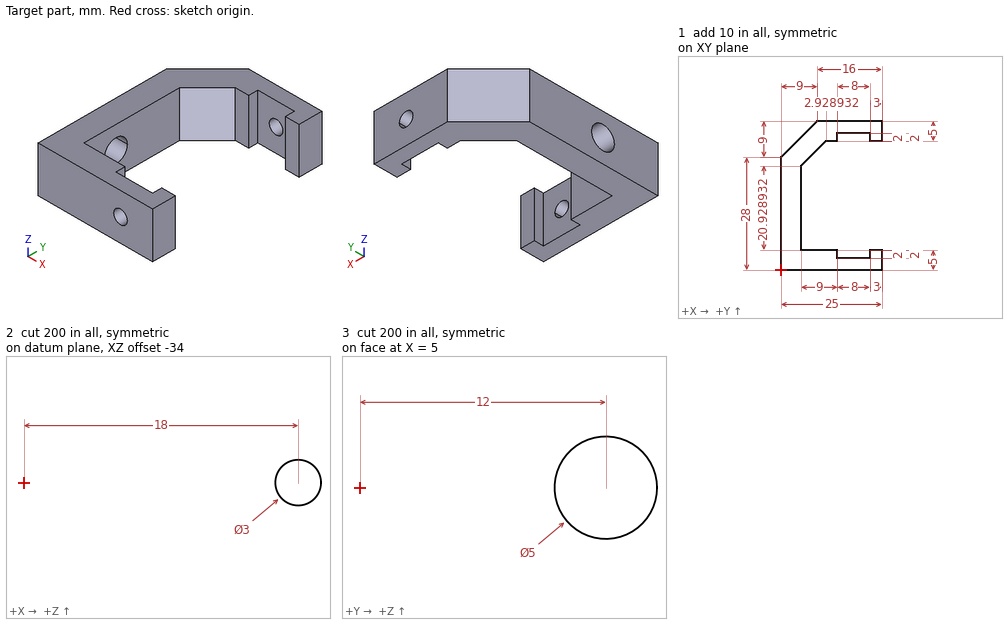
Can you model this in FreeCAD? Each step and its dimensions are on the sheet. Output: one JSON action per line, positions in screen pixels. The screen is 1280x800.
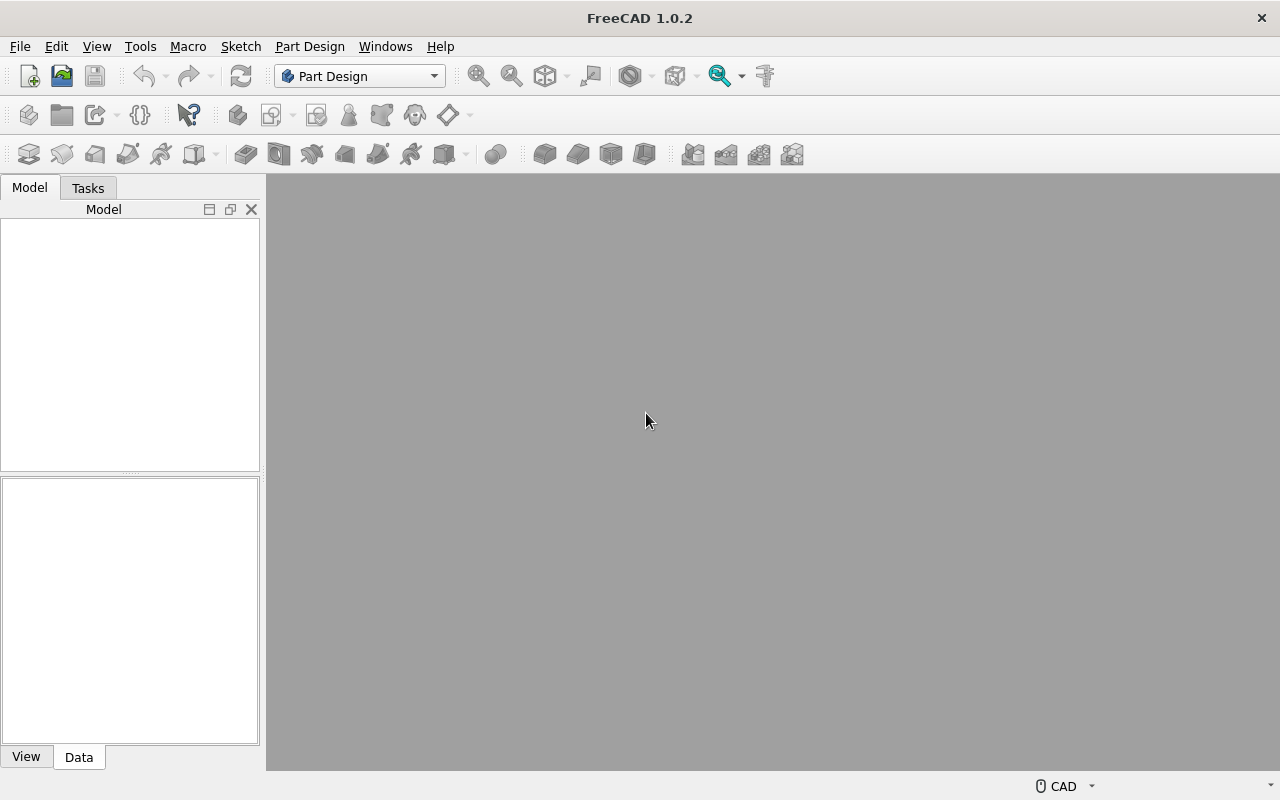
{"action": "left_click", "coordinate": [29, 76]}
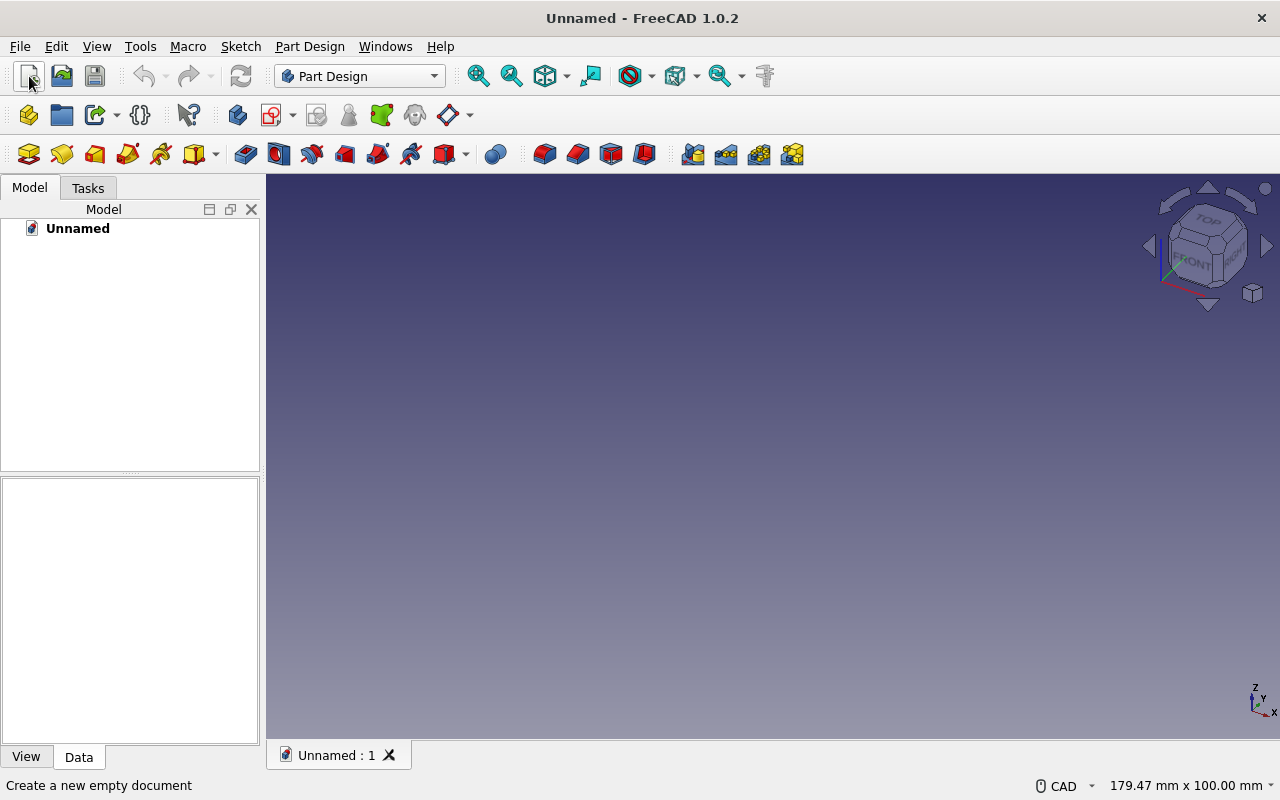
{"action": "left_click", "coordinate": [270, 116]}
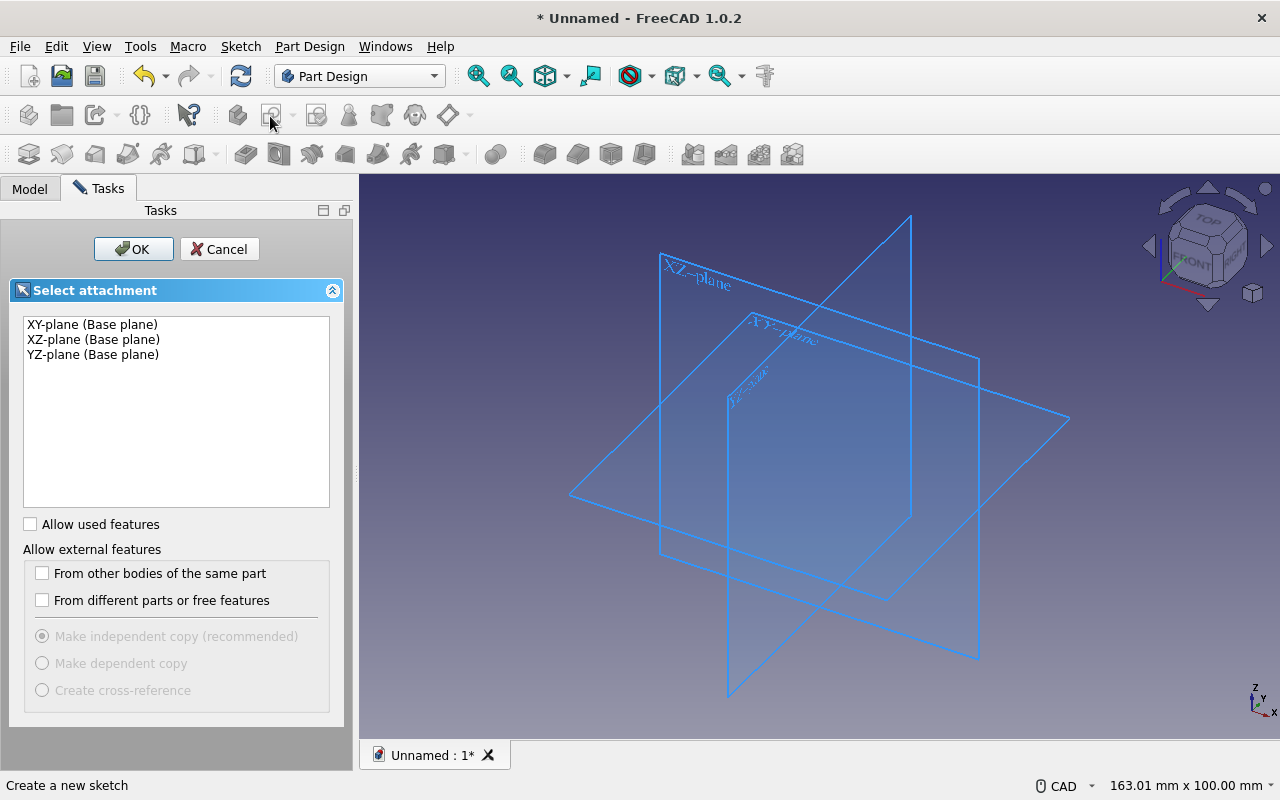
{"action": "left_click", "coordinate": [84, 324]}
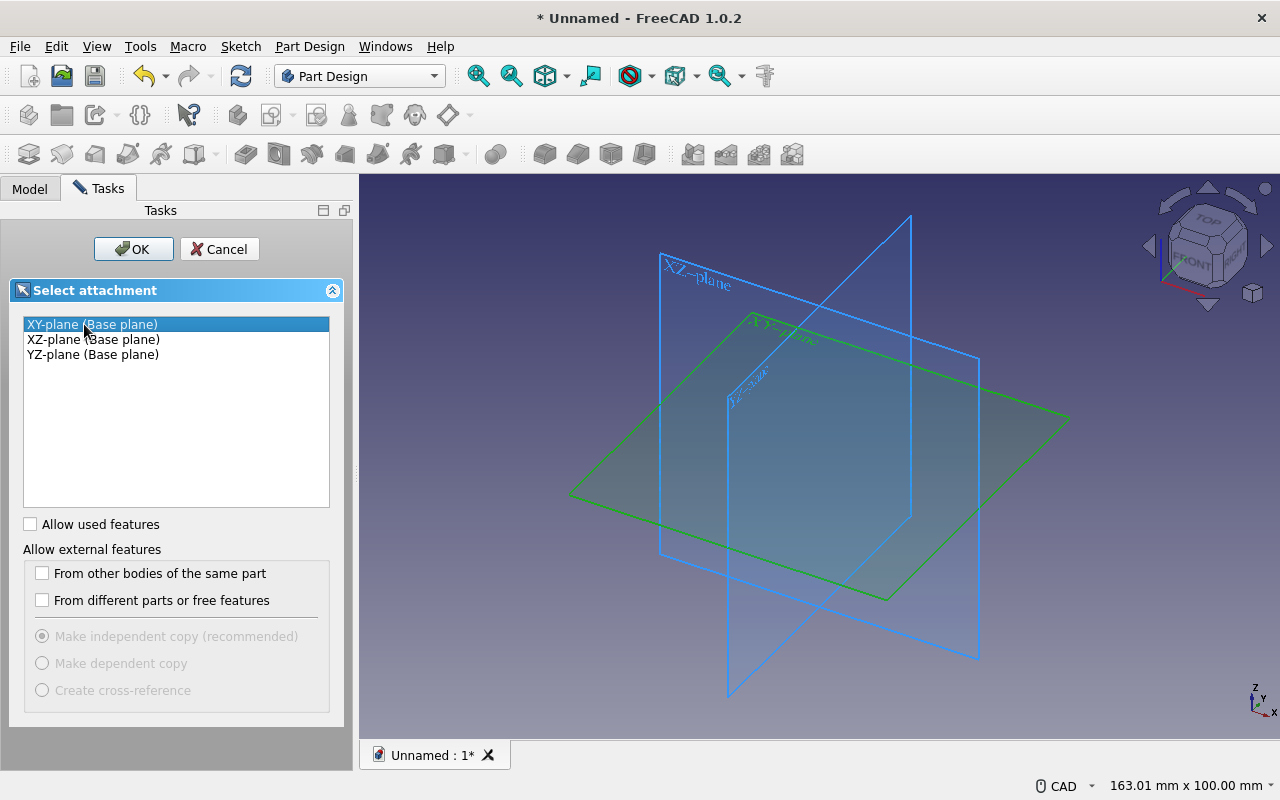
{"action": "left_click", "coordinate": [134, 249]}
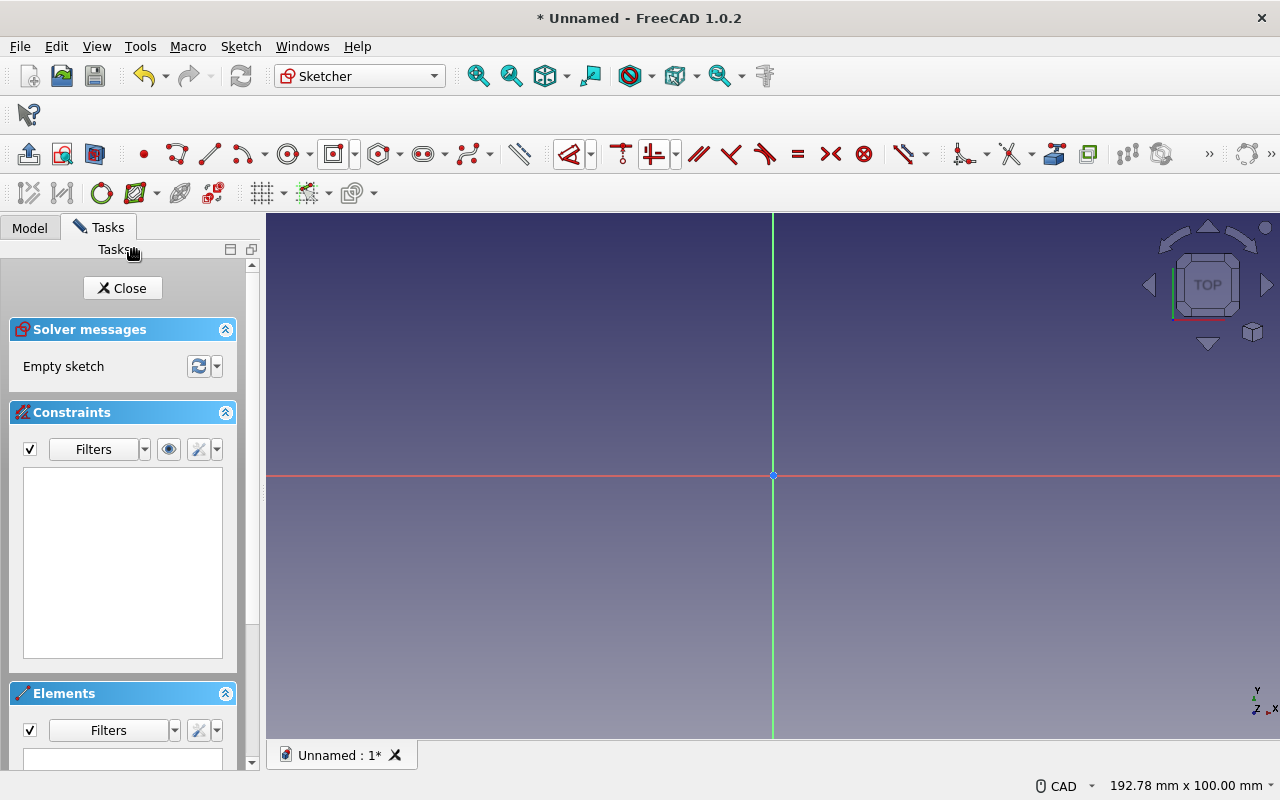
{"action": "scroll", "coordinate": [1002, 260], "scroll_direction": "up", "scroll_amount": 3}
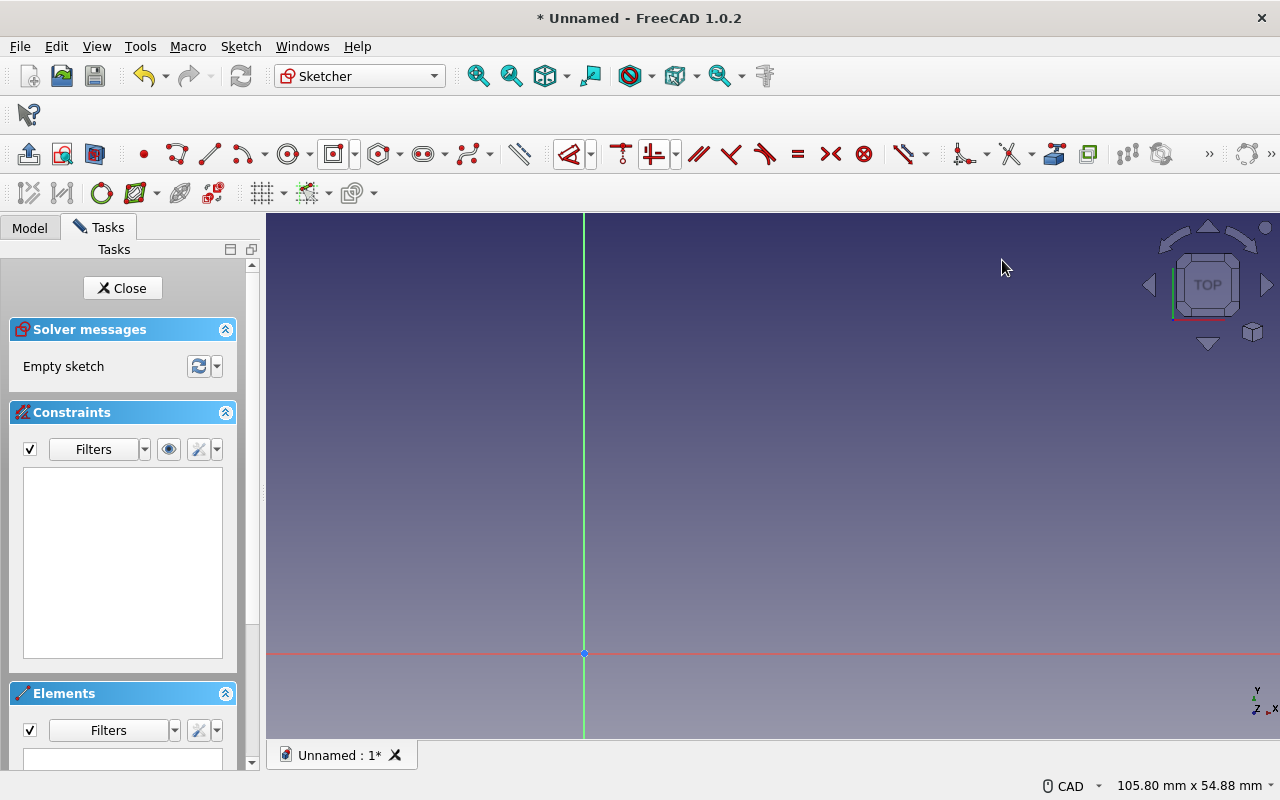
{"action": "left_click", "coordinate": [177, 154]}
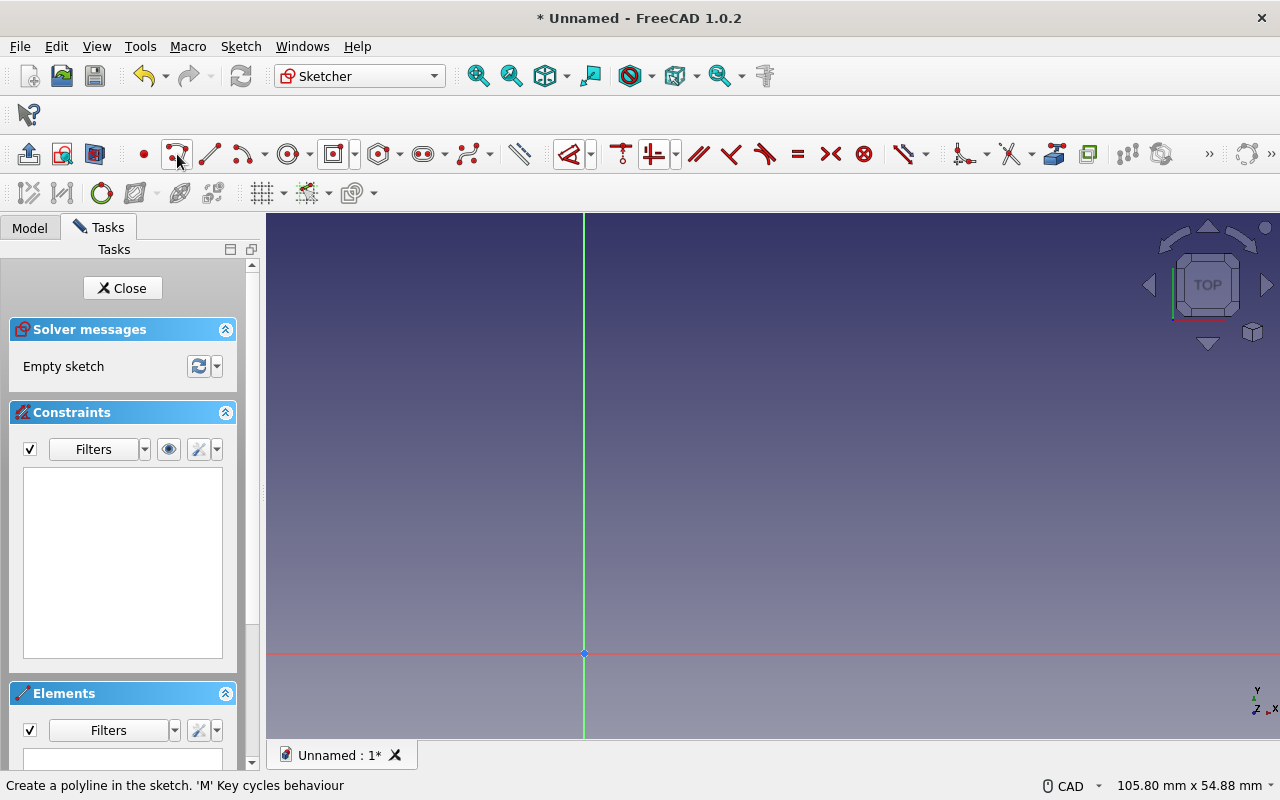
{"action": "left_click", "coordinate": [584, 654]}
{"action": "left_click", "coordinate": [824, 645]}
{"action": "left_click", "coordinate": [824, 606]}
{"action": "left_click", "coordinate": [795, 606]}
{"action": "left_click", "coordinate": [795, 625]}
{"action": "left_click", "coordinate": [718, 625]}
{"action": "left_click", "coordinate": [718, 606]}
{"action": "left_click", "coordinate": [632, 606]}
{"action": "left_click", "coordinate": [632, 405]}
{"action": "left_click", "coordinate": [690, 347]}
{"action": "left_click", "coordinate": [718, 347]}
{"action": "left_click", "coordinate": [718, 328]}
{"action": "left_click", "coordinate": [795, 328]}
{"action": "left_click", "coordinate": [795, 347]}
{"action": "left_click", "coordinate": [824, 347]}
{"action": "left_click", "coordinate": [824, 299]}
{"action": "left_click", "coordinate": [670, 299]}
{"action": "left_click", "coordinate": [593, 385]}
{"action": "left_click", "coordinate": [584, 654]}
{"action": "key", "text": "Escape"}
{"action": "key", "text": "Escape"}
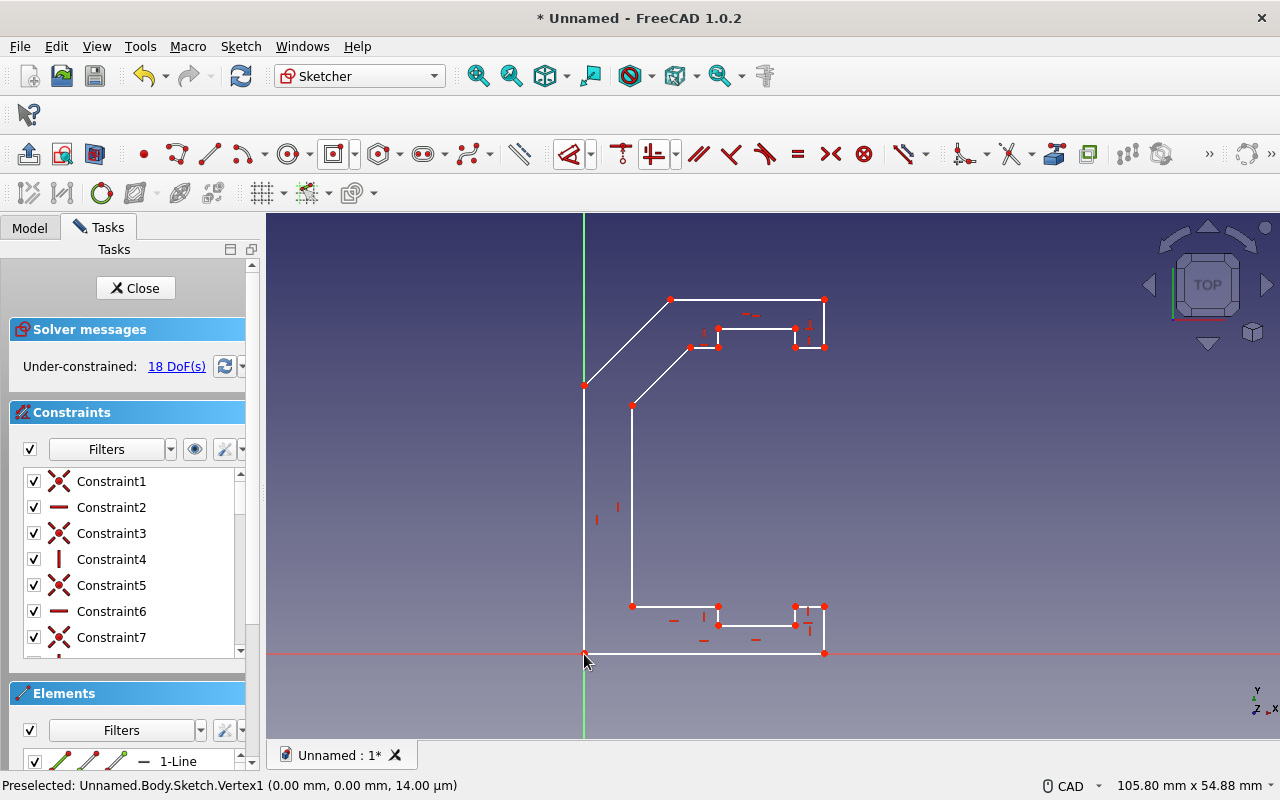
{"action": "key", "text": "d"}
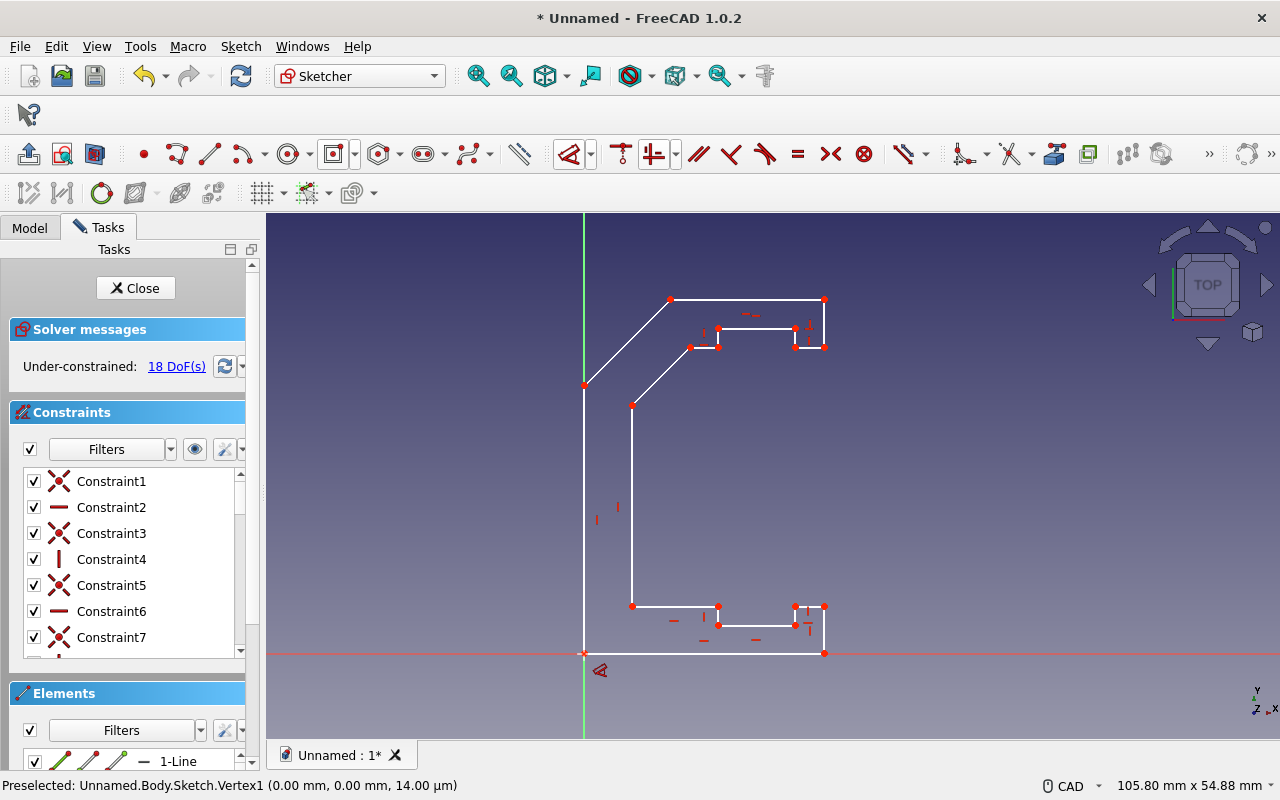
{"action": "left_click", "coordinate": [824, 640]}
{"action": "left_click", "coordinate": [858, 630]}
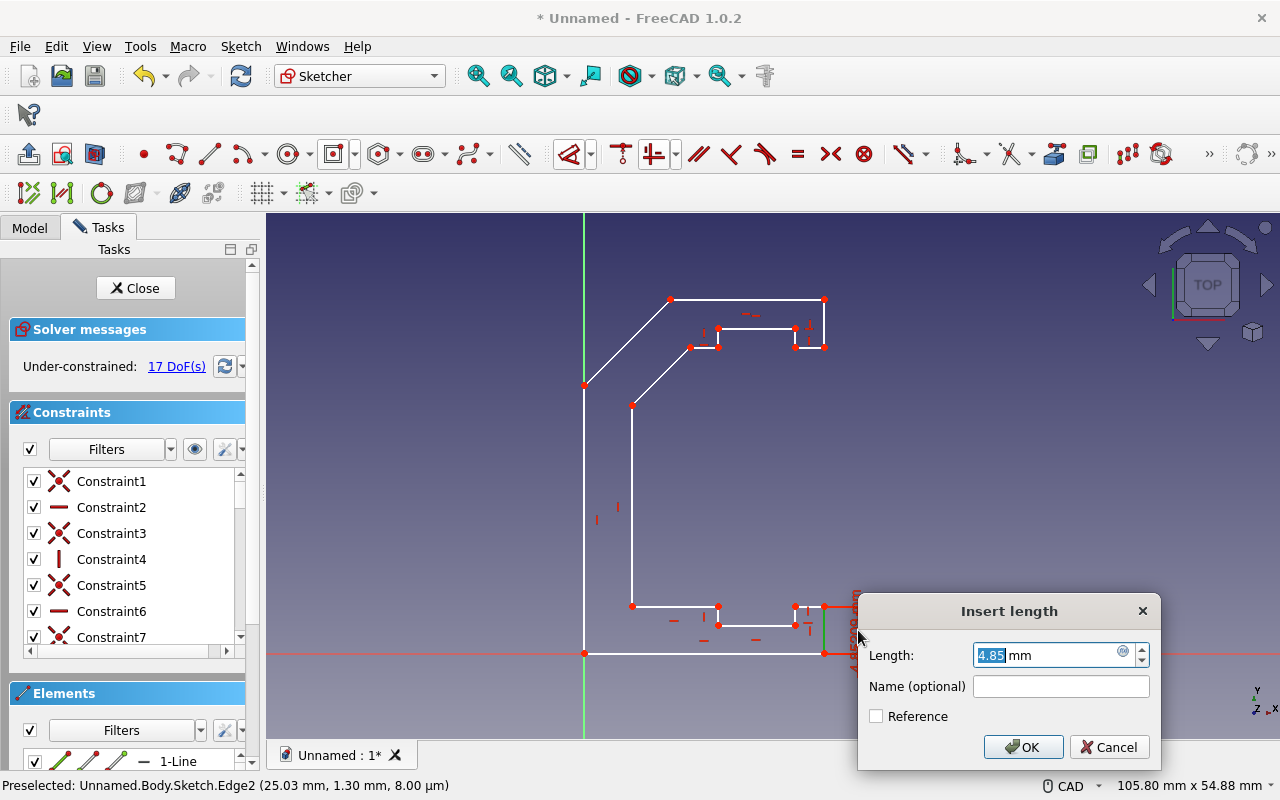
{"action": "type", "text": "5"}
{"action": "key", "text": "Return"}